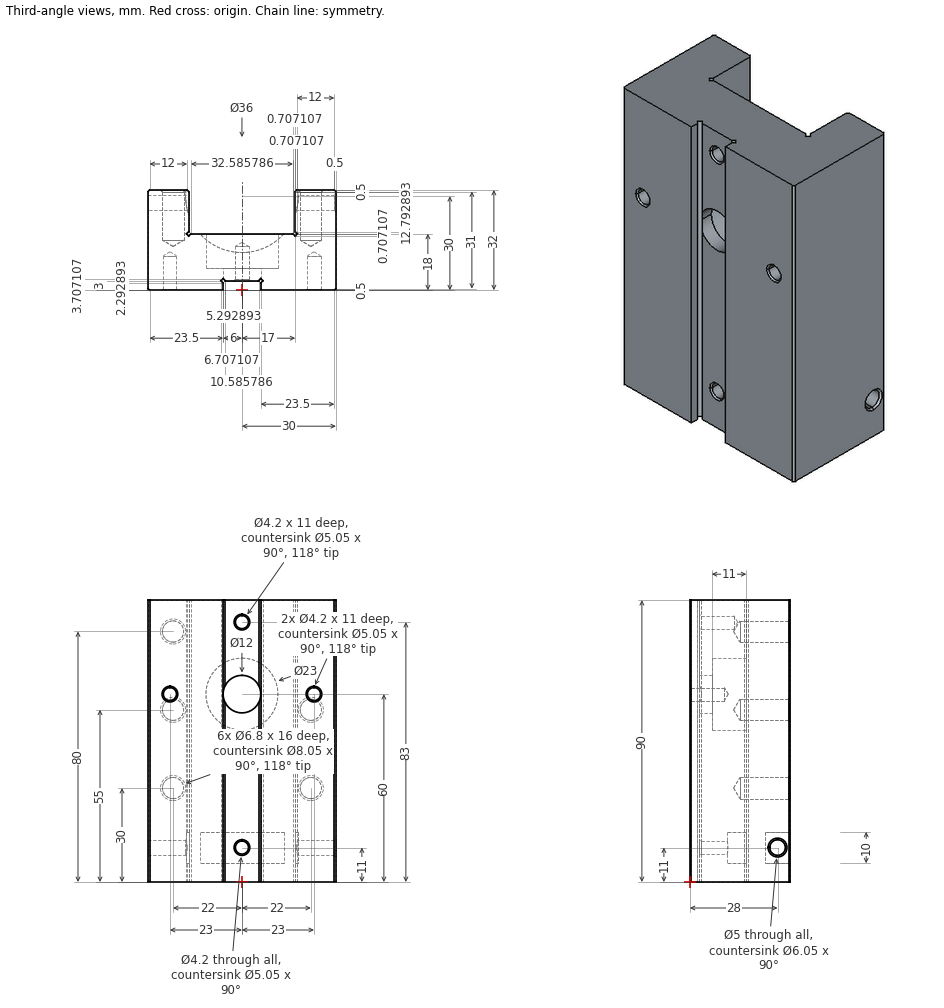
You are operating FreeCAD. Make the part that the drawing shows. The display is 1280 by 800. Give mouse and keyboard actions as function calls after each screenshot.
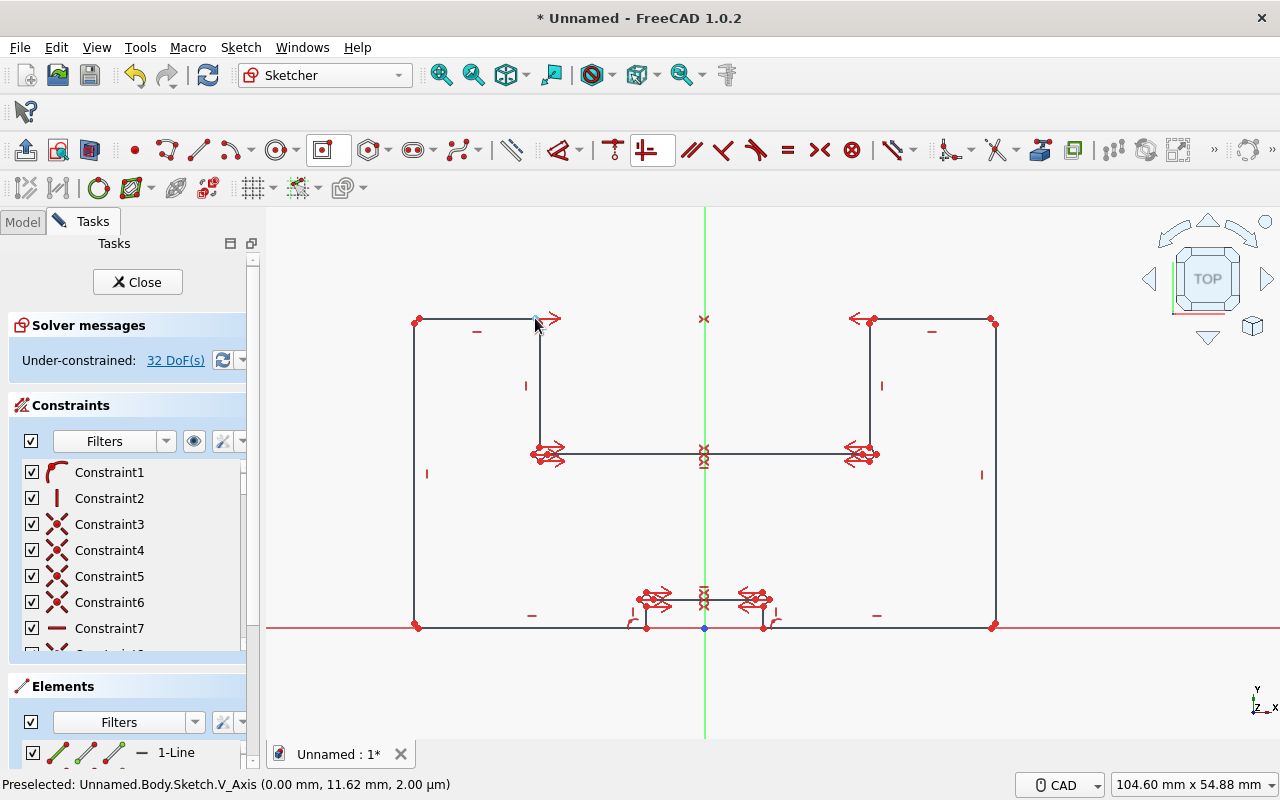
scroll(996, 324, up, 3)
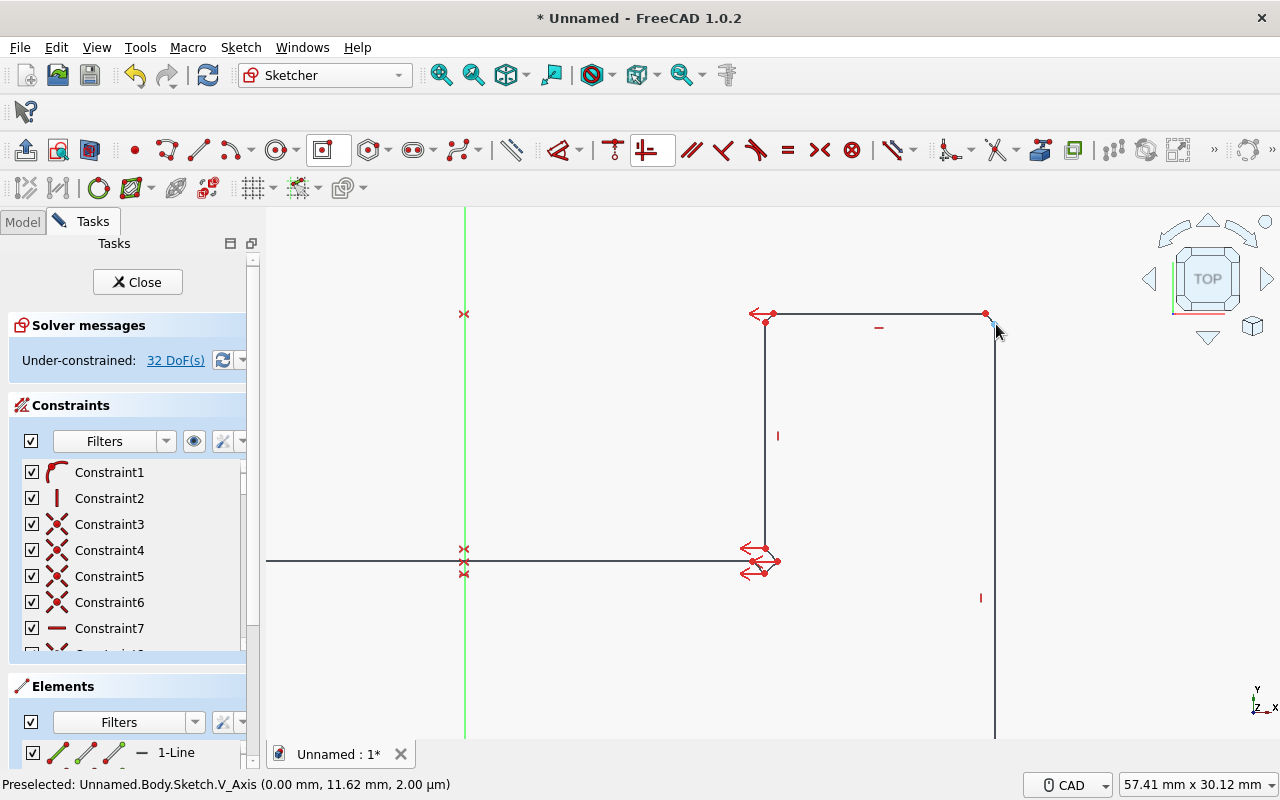
click(995, 324)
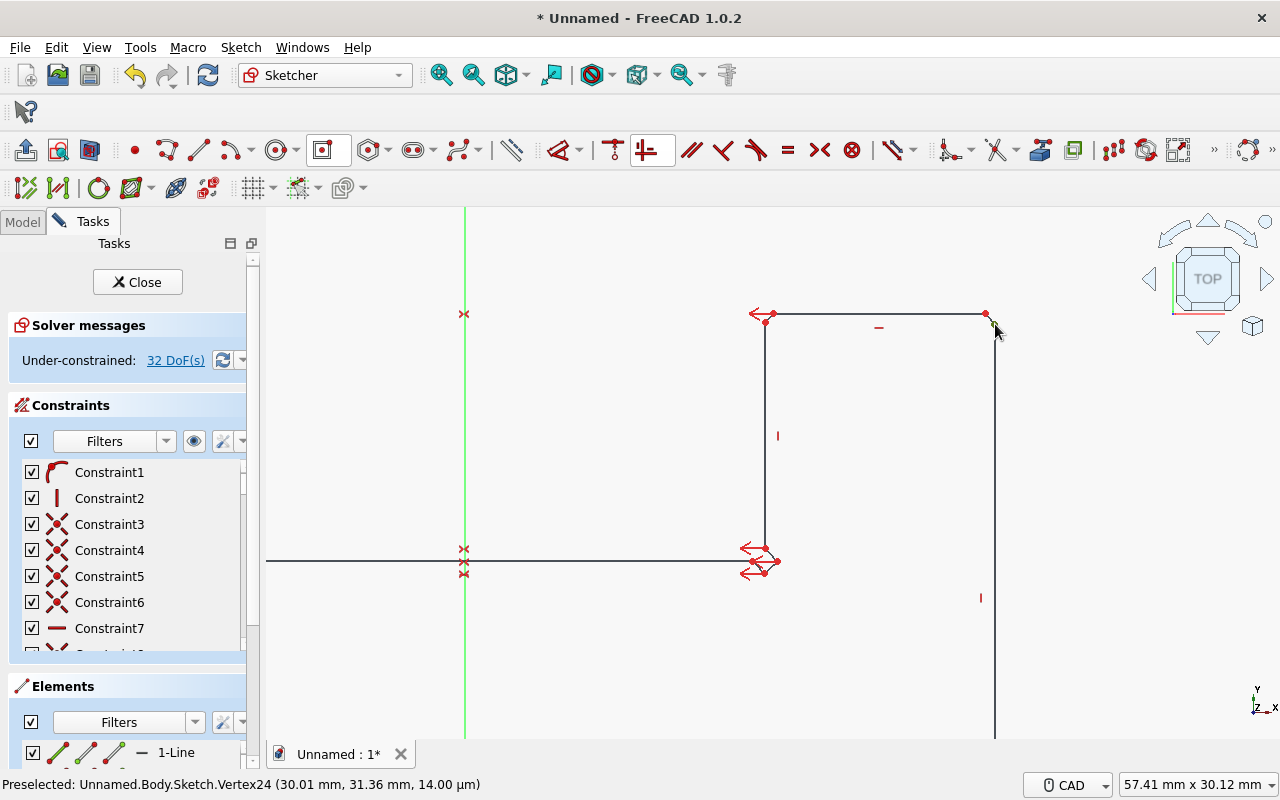
scroll(996, 324, down, 3)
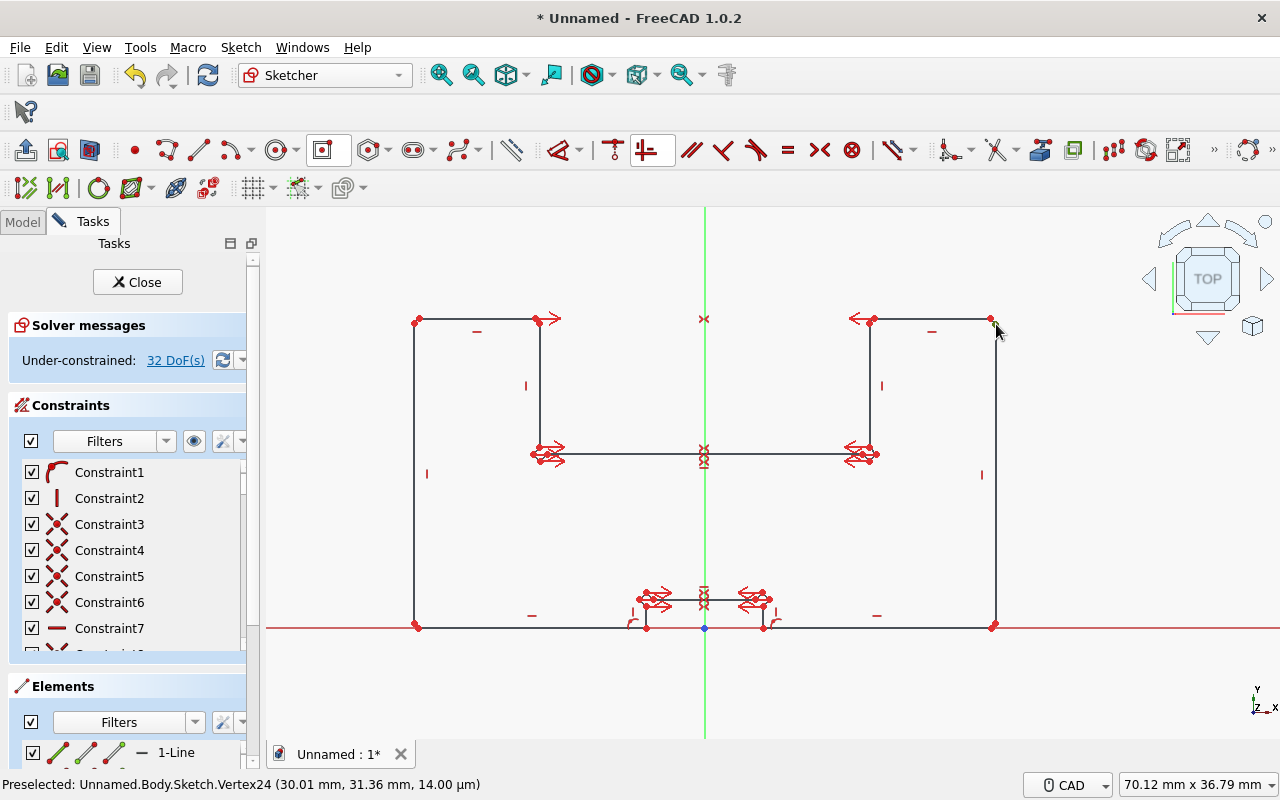
scroll(414, 324, up, 3)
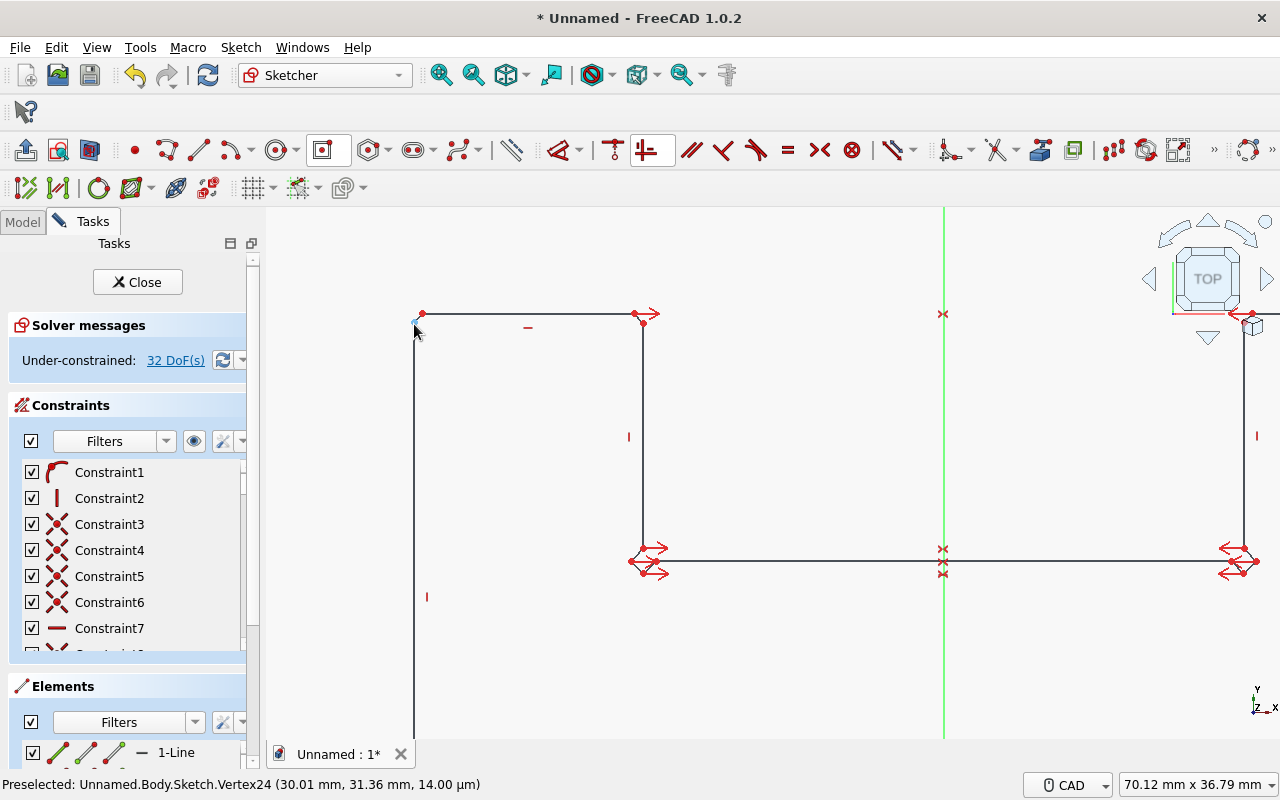
click(414, 323)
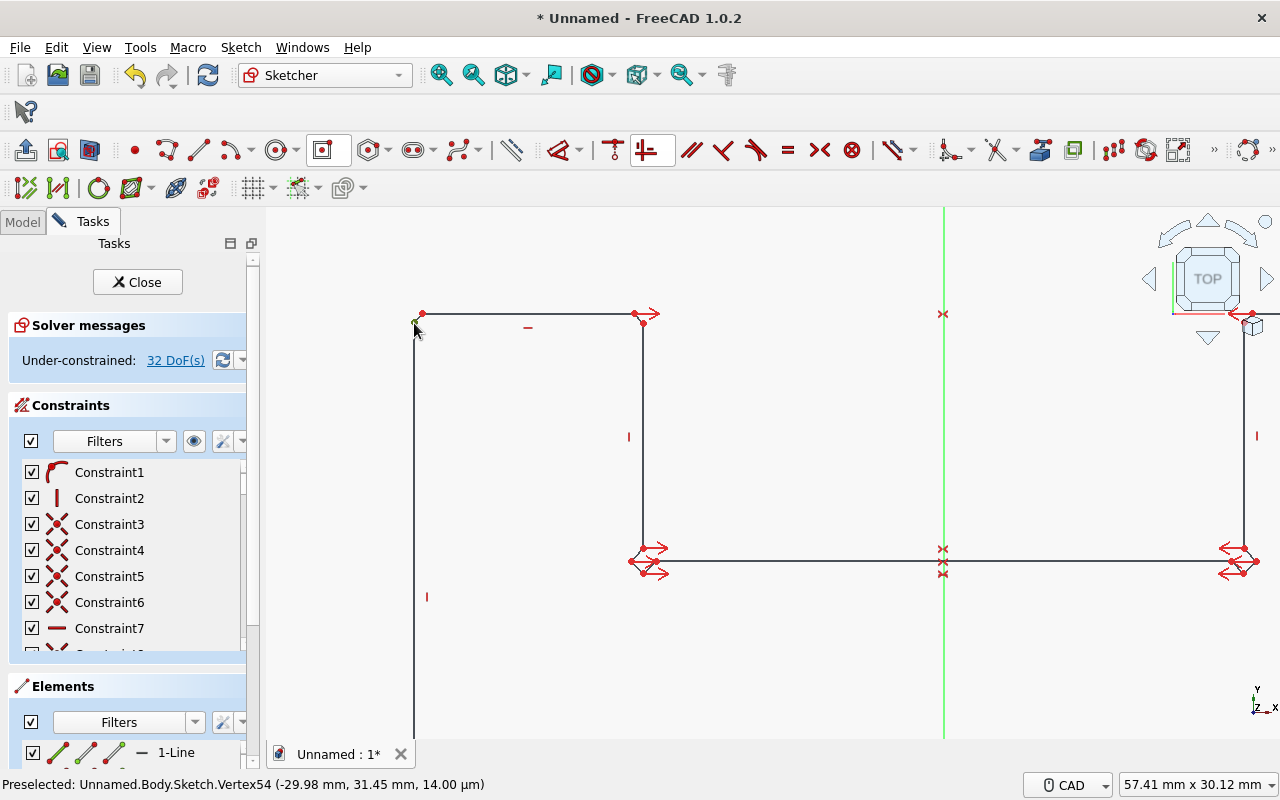
click(944, 677)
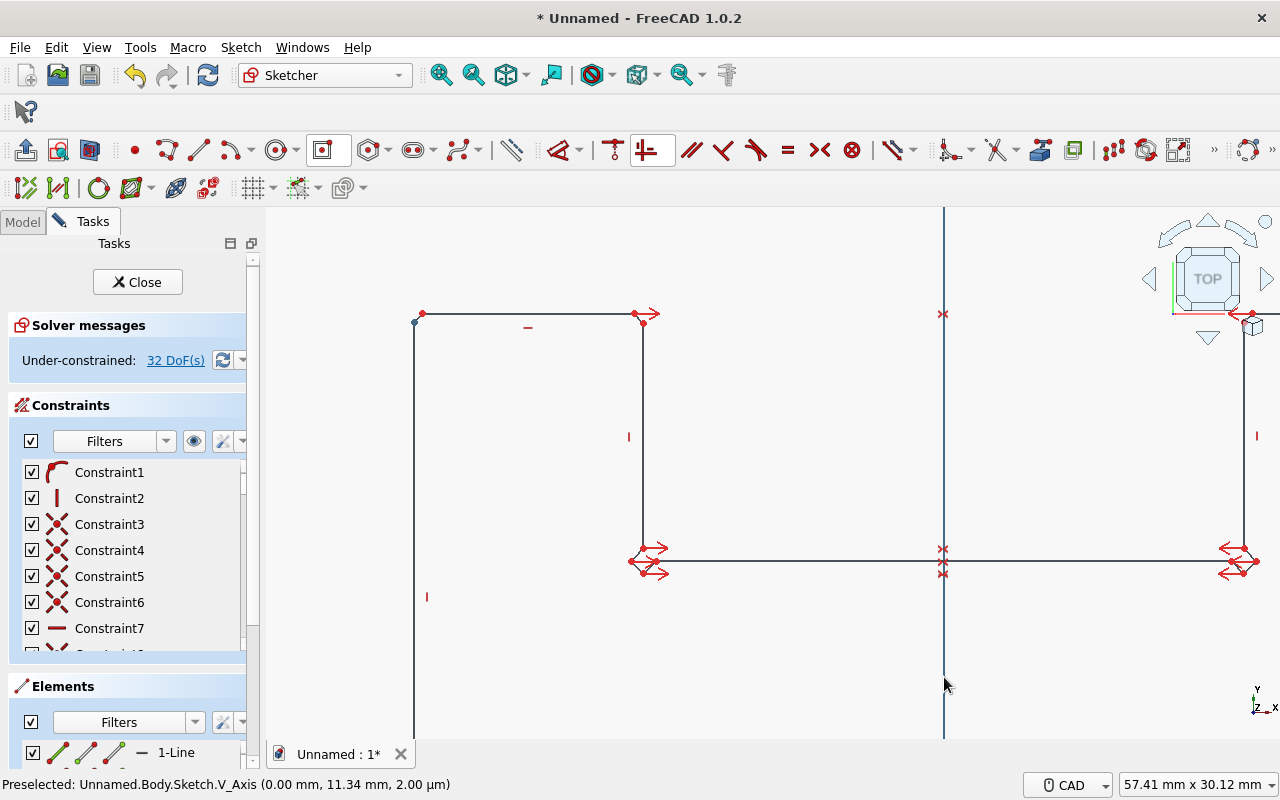
click(820, 150)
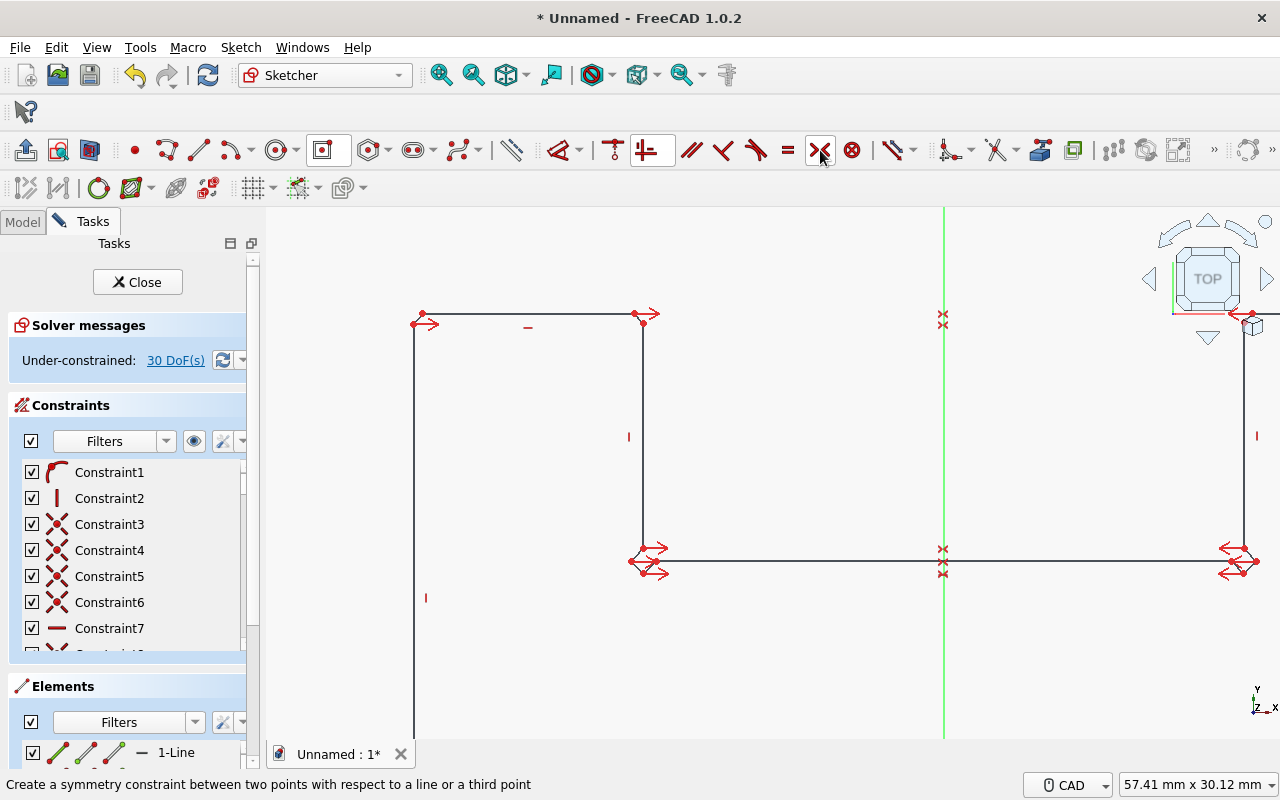
click(558, 150)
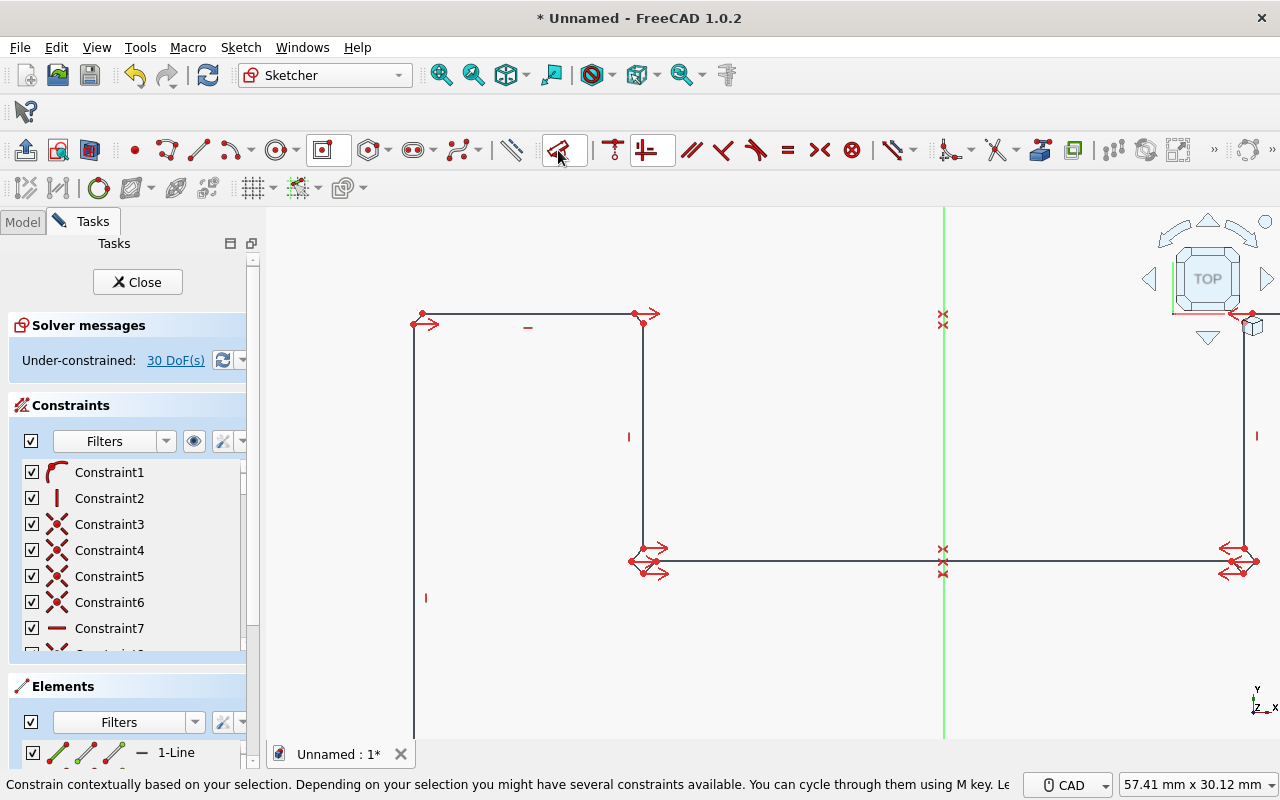
scroll(414, 324, down, 3)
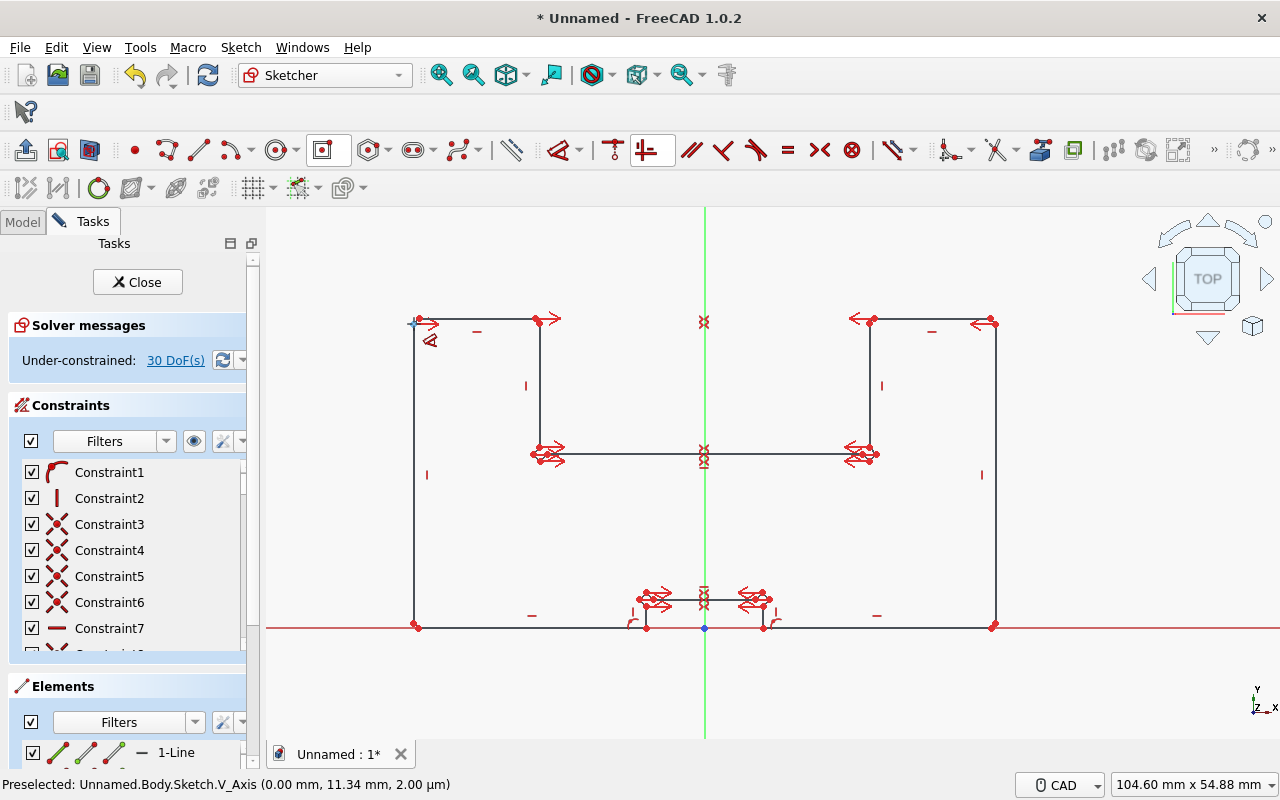
click(996, 534)
click(1030, 474)